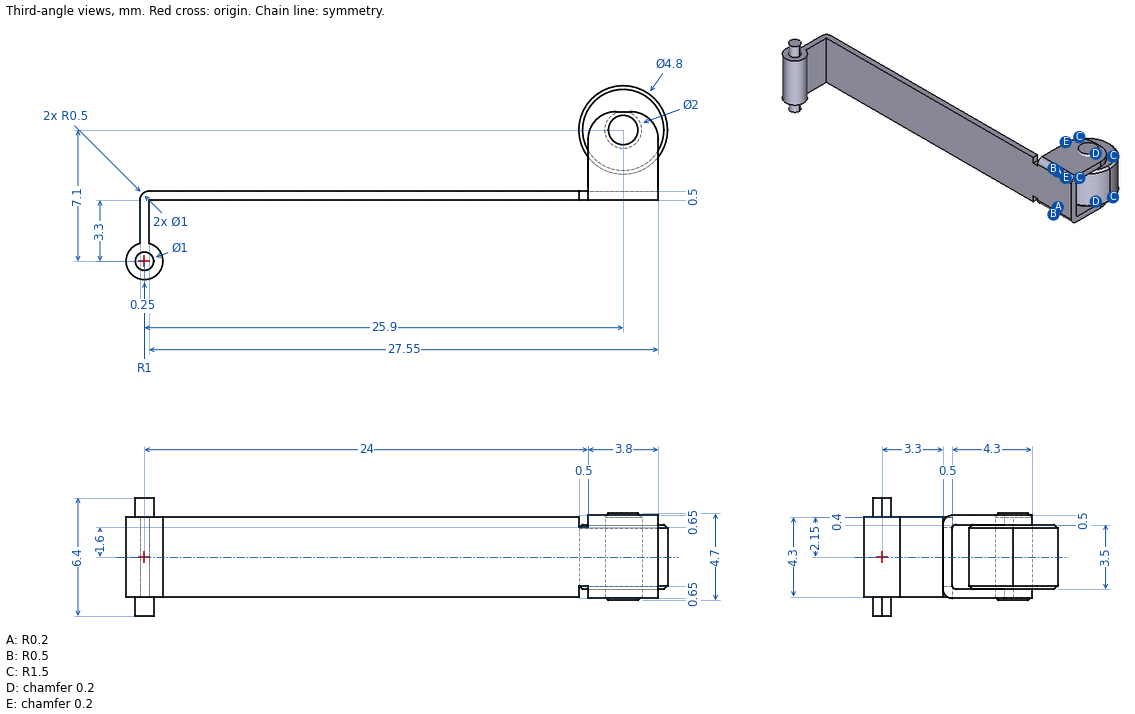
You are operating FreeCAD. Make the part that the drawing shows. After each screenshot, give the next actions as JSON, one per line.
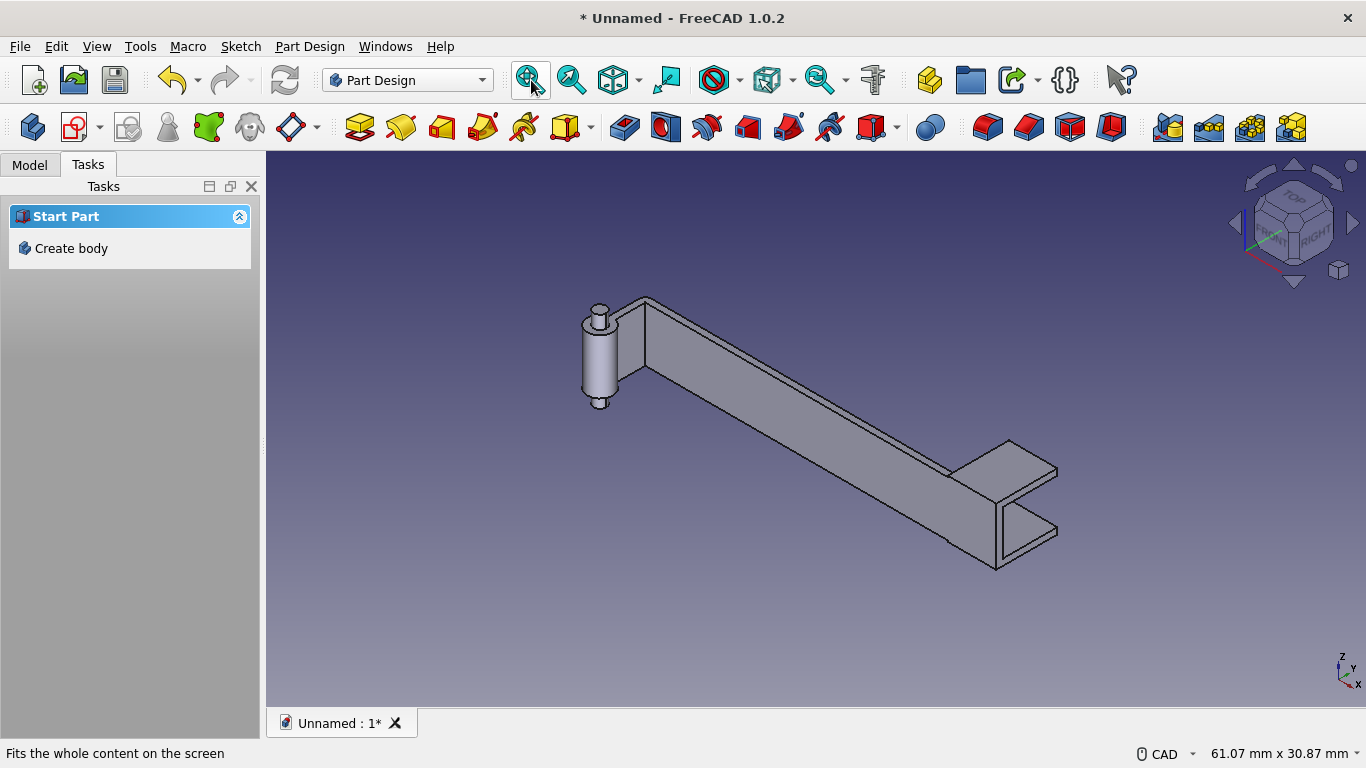
{"action": "key", "text": "2"}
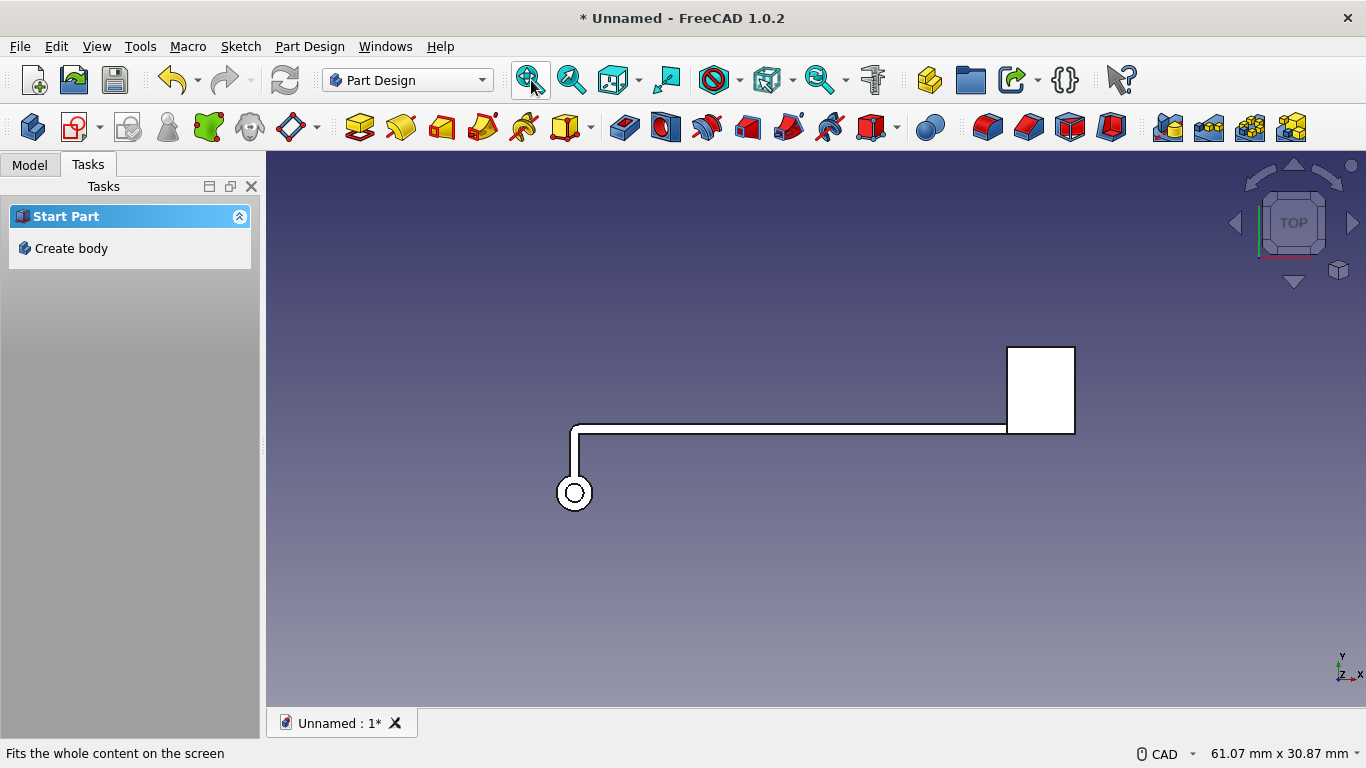
{"action": "key", "text": "0"}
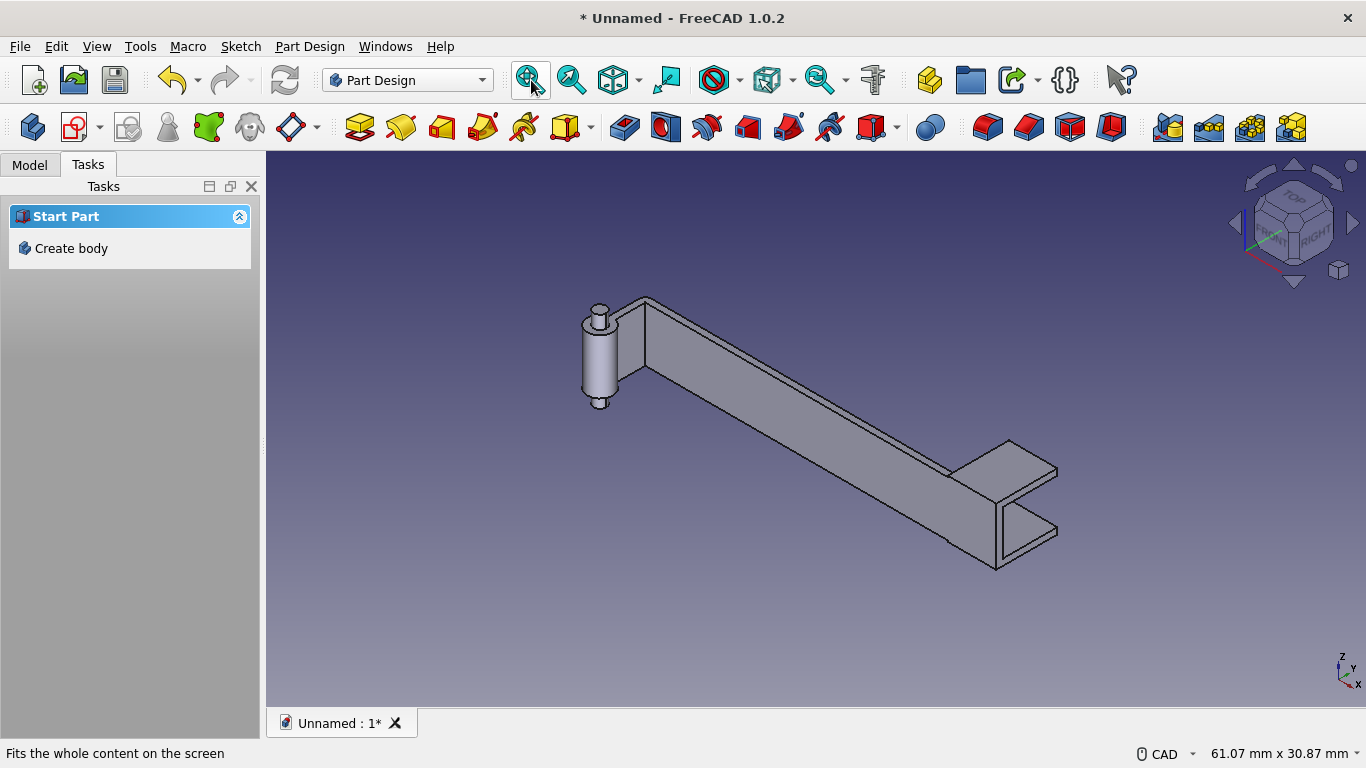
{"action": "key", "text": "1"}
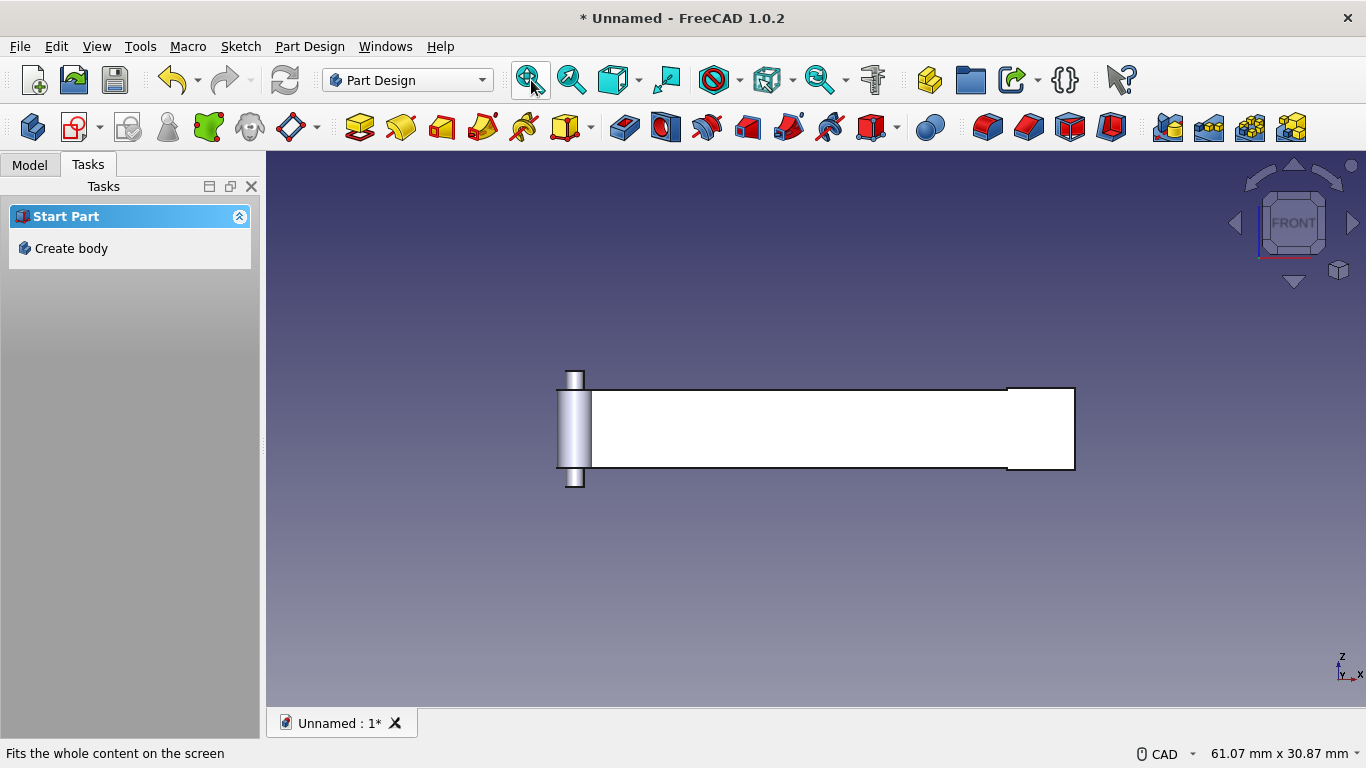
{"action": "key", "text": "3"}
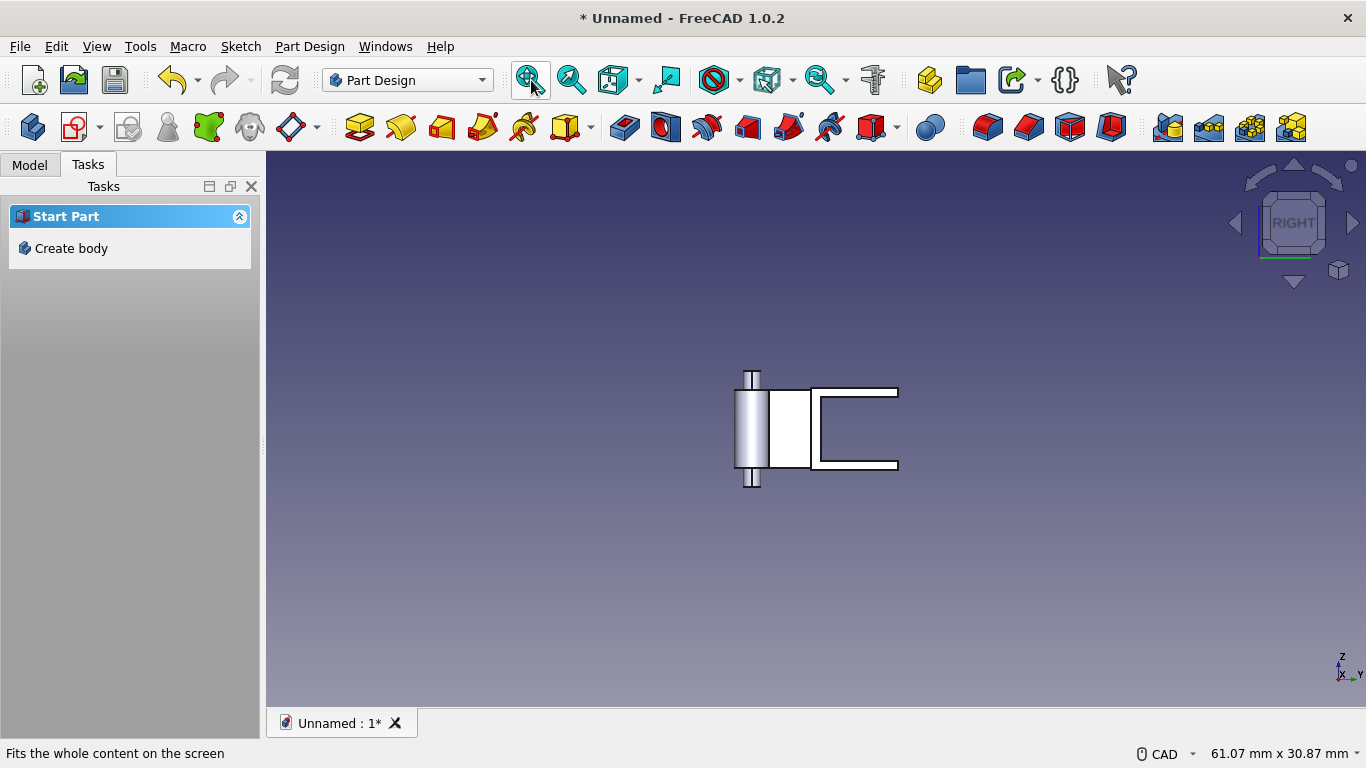
{"action": "key", "text": "v f"}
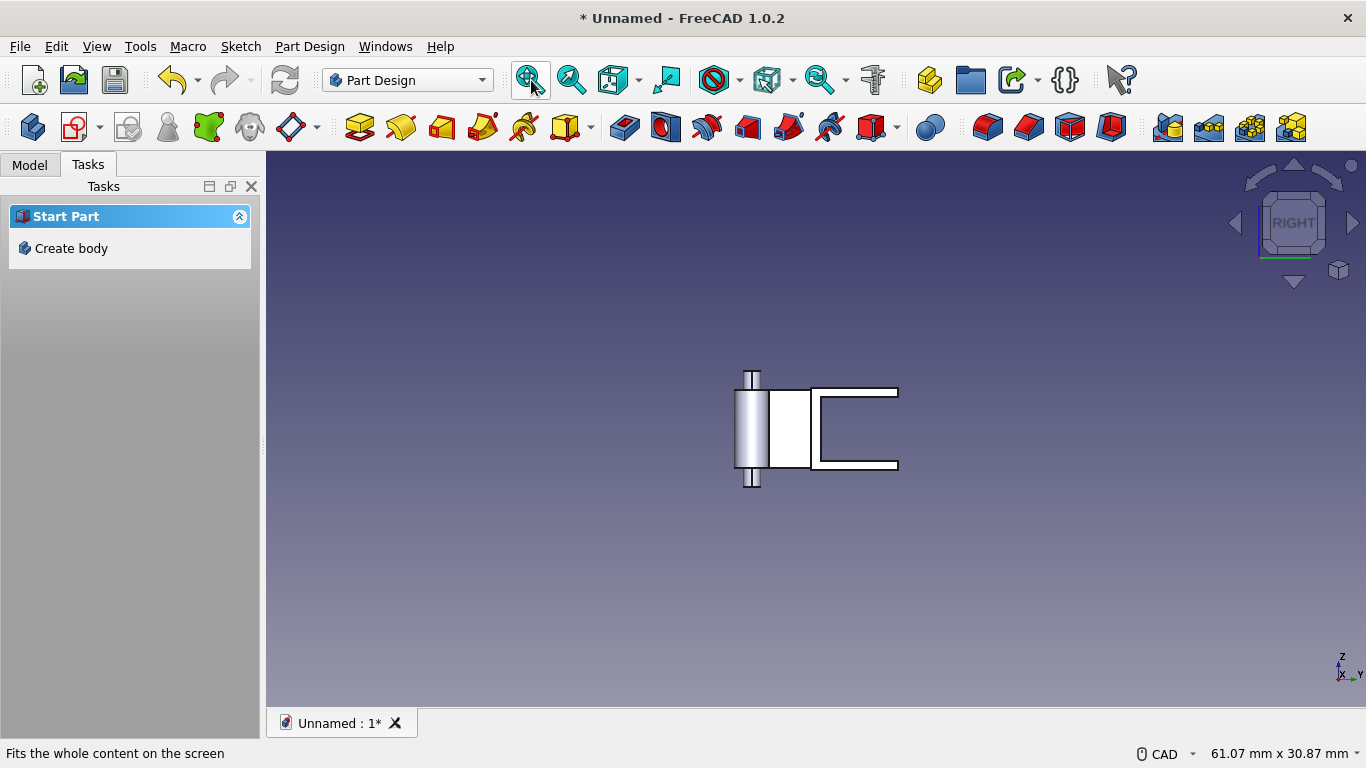
{"action": "key", "text": "5"}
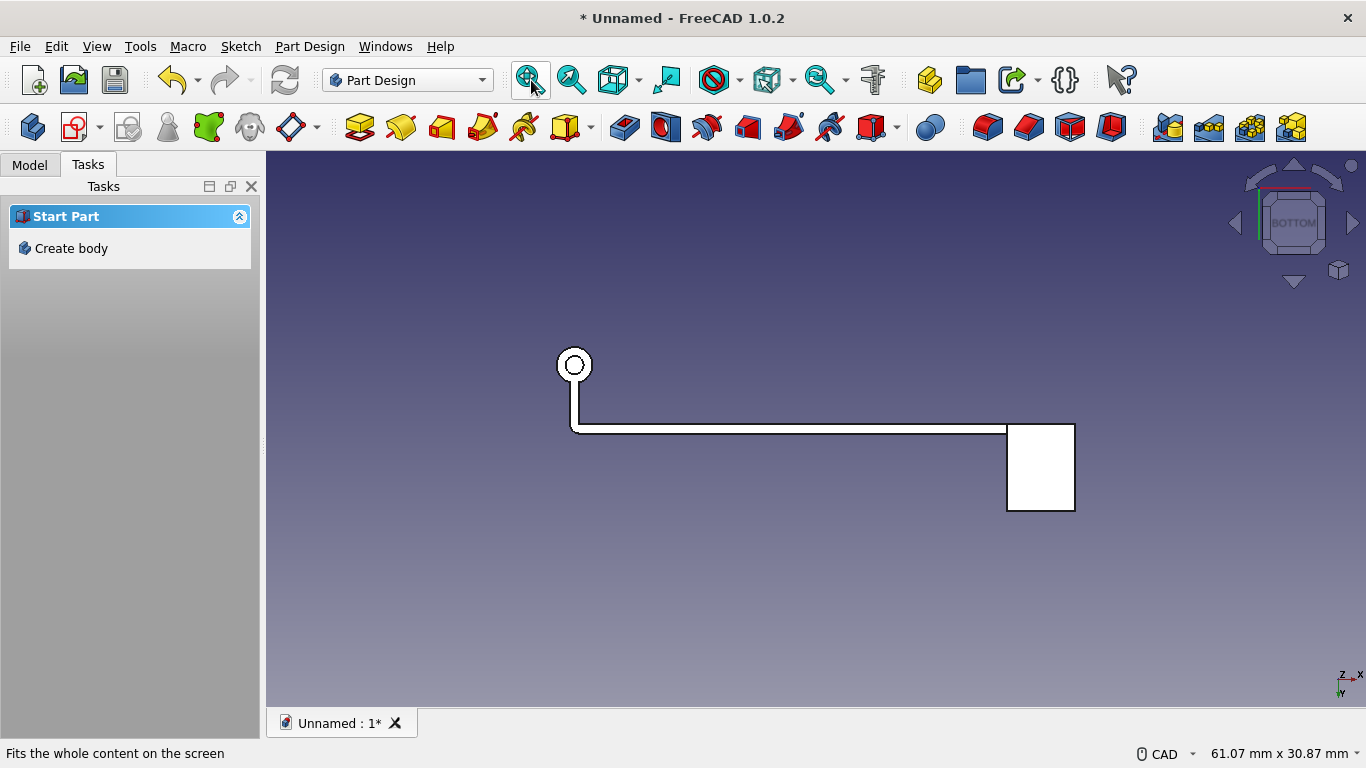
{"action": "key", "text": "4"}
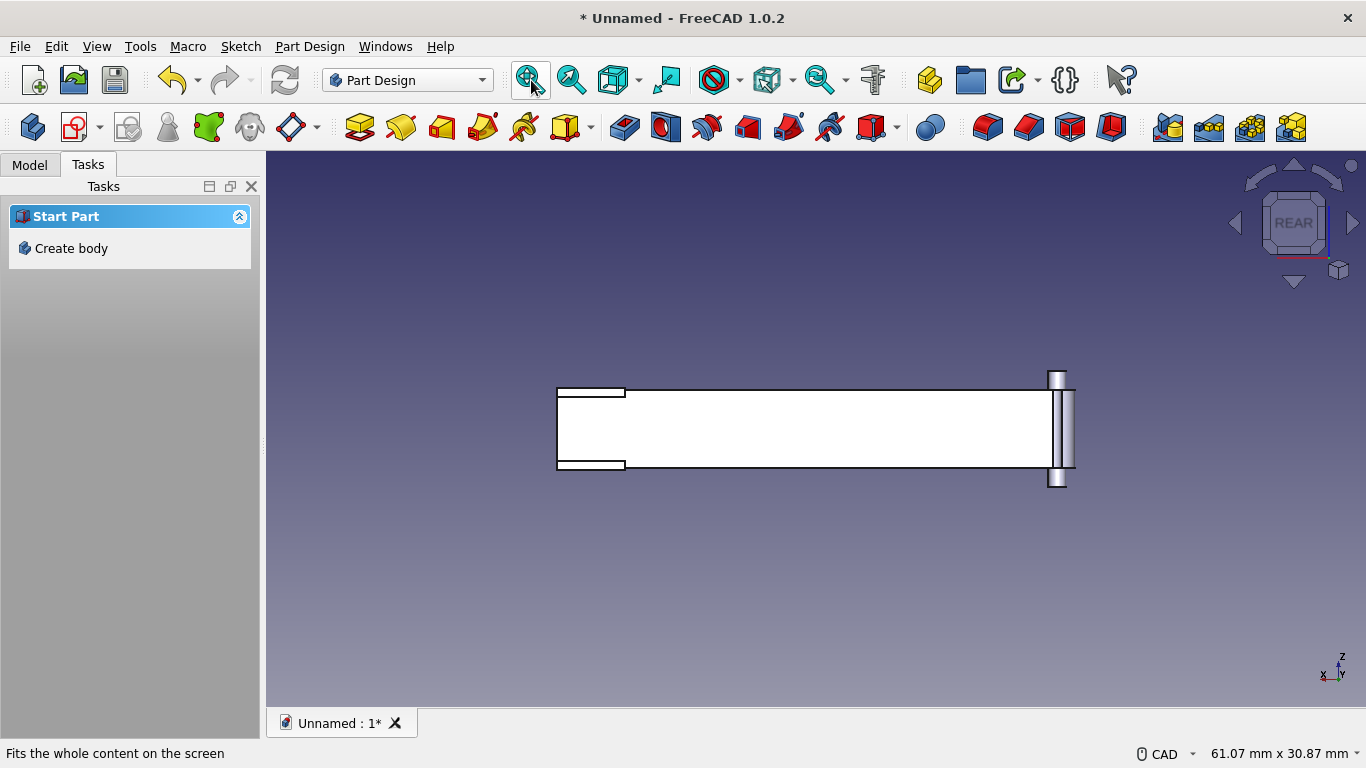
{"action": "key", "text": "6"}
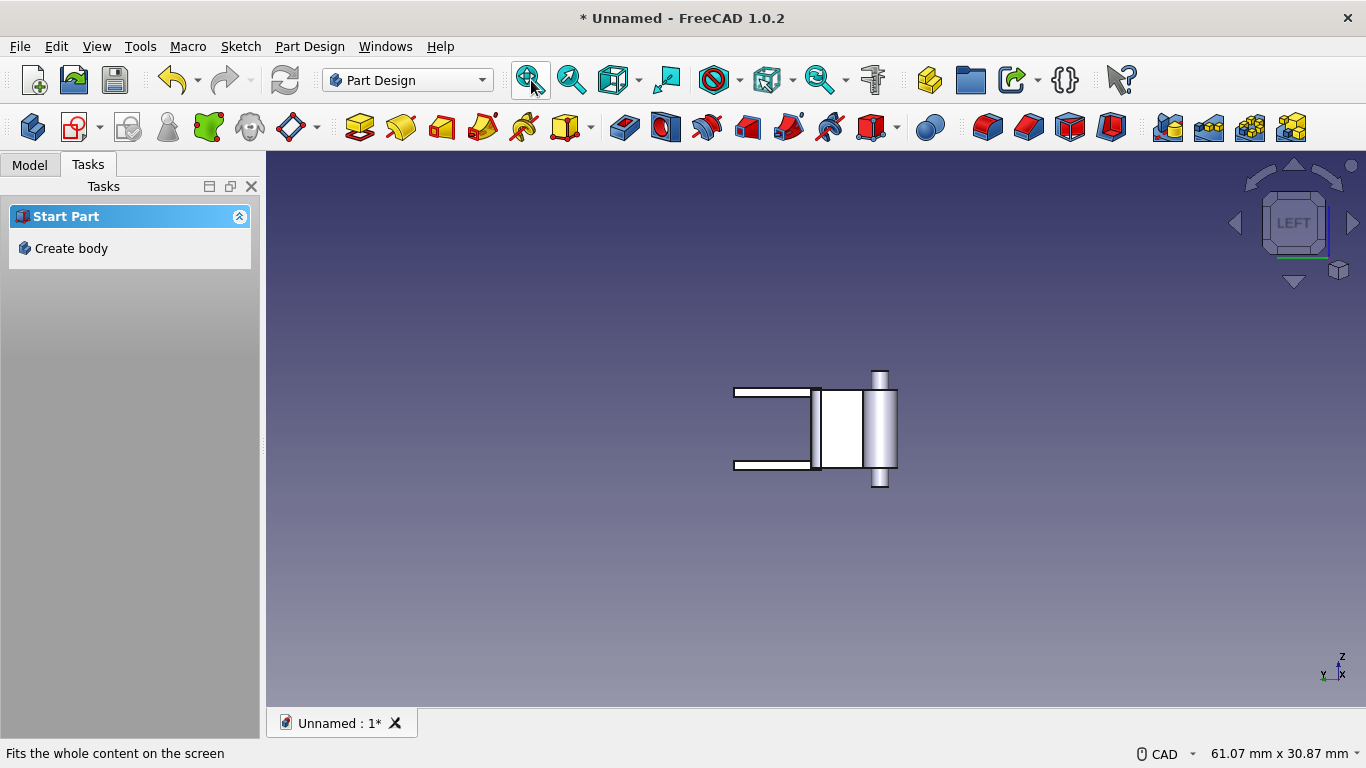
{"action": "left_click", "coordinate": [531, 80]}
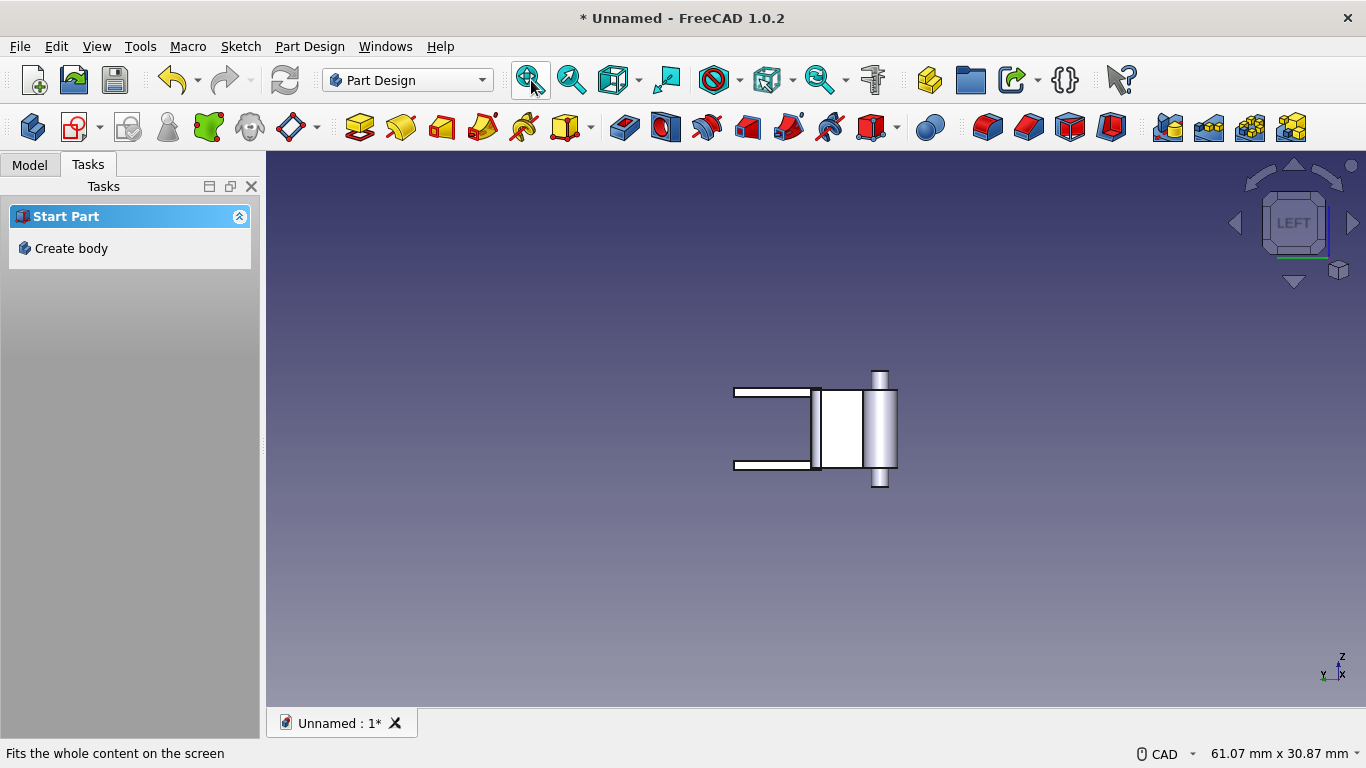
{"action": "key", "text": "v 3"}